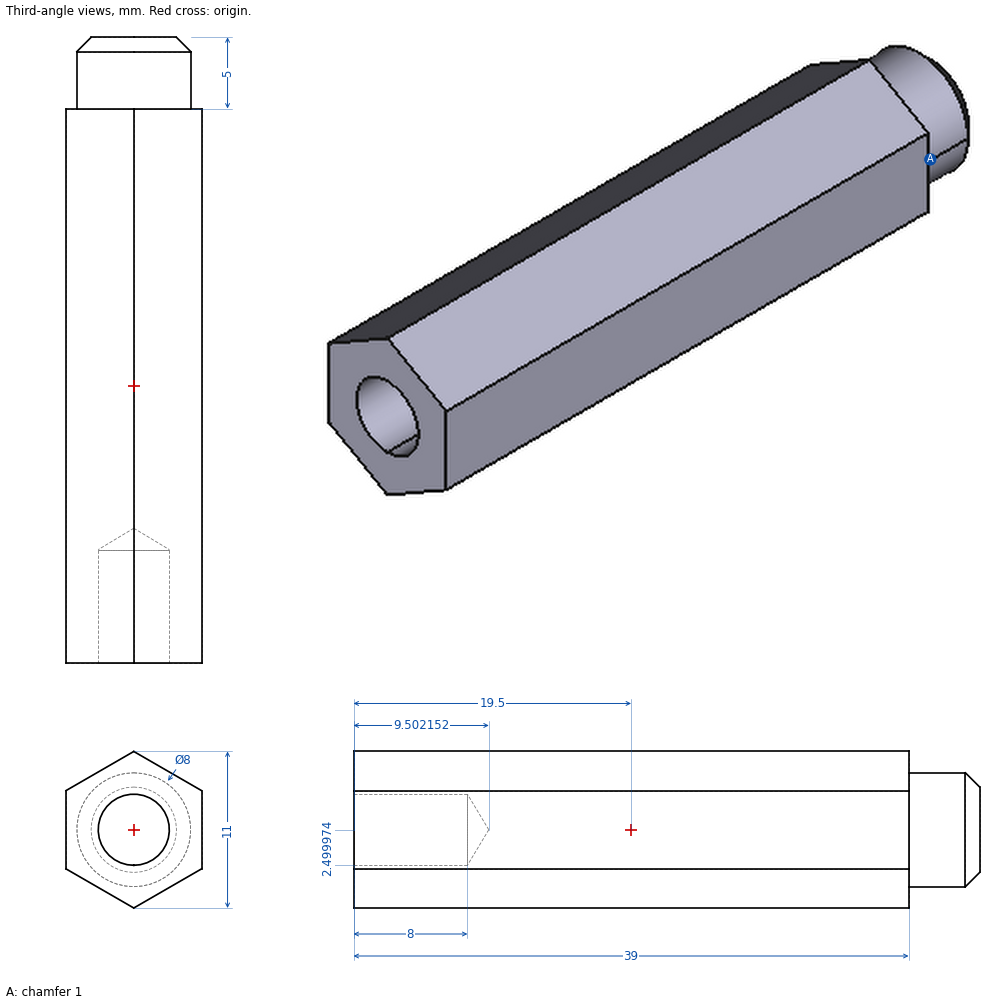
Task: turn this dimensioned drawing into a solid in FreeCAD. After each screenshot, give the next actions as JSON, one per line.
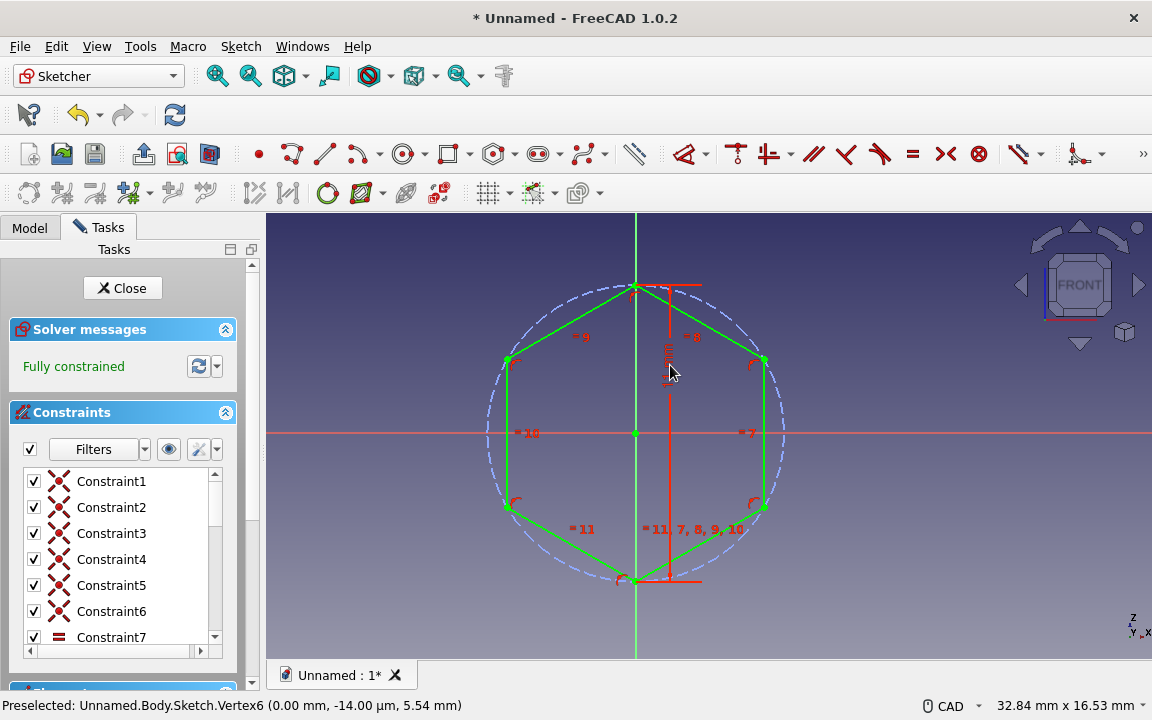
{"action": "left_click", "coordinate": [123, 288]}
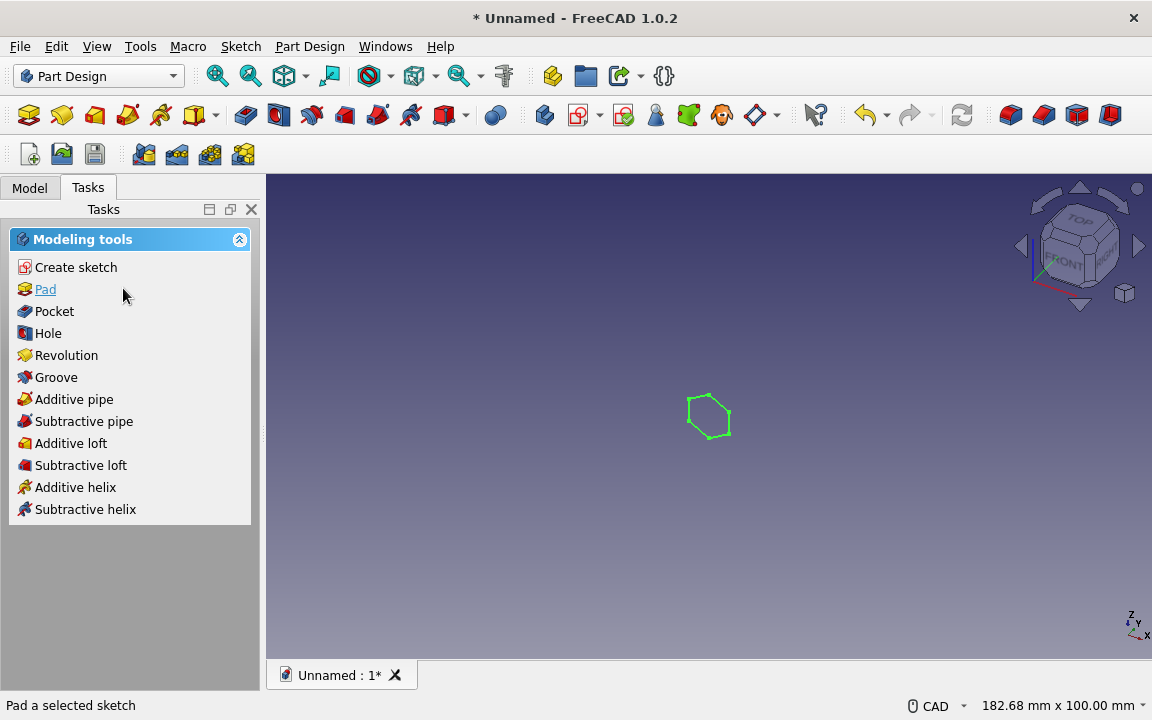
{"action": "left_click", "coordinate": [29, 116]}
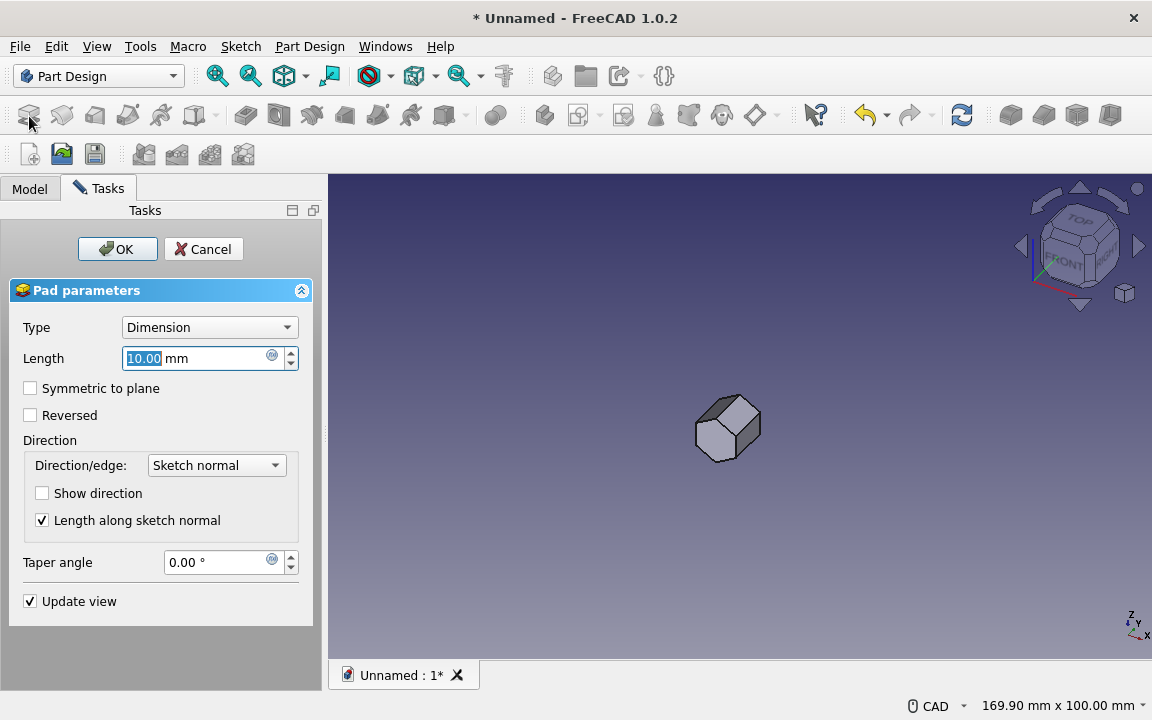
{"action": "type", "text": "39"}
{"action": "key", "text": "Tab"}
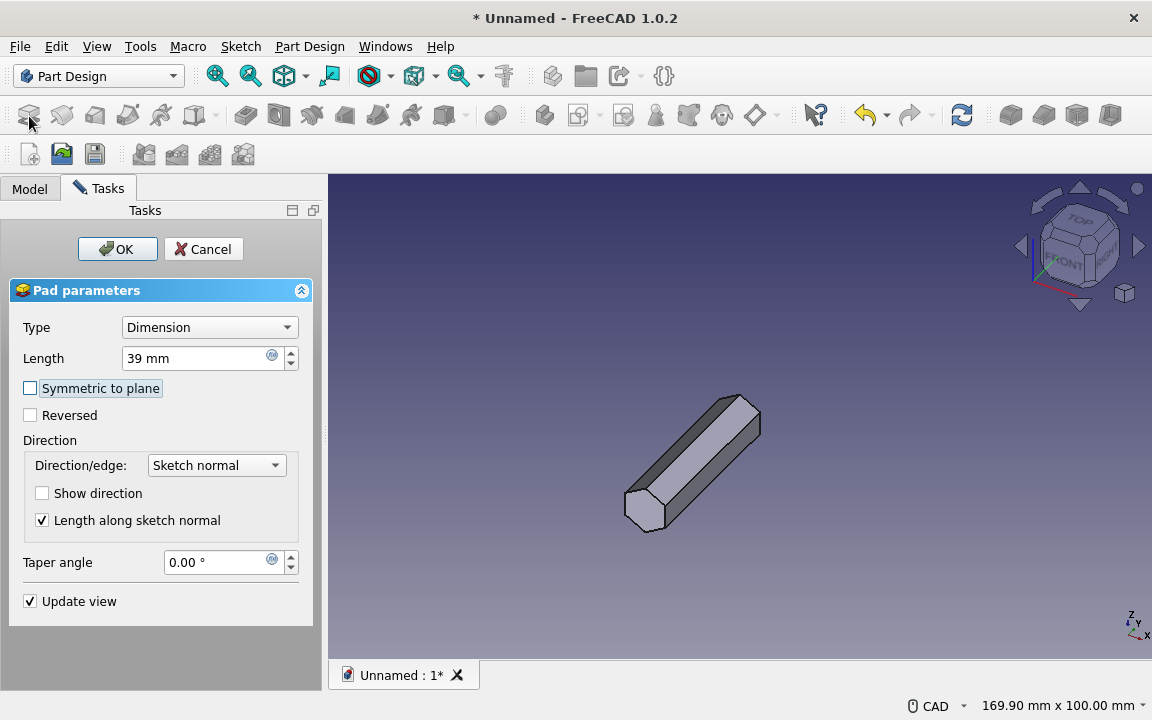
{"action": "left_click", "coordinate": [31, 388]}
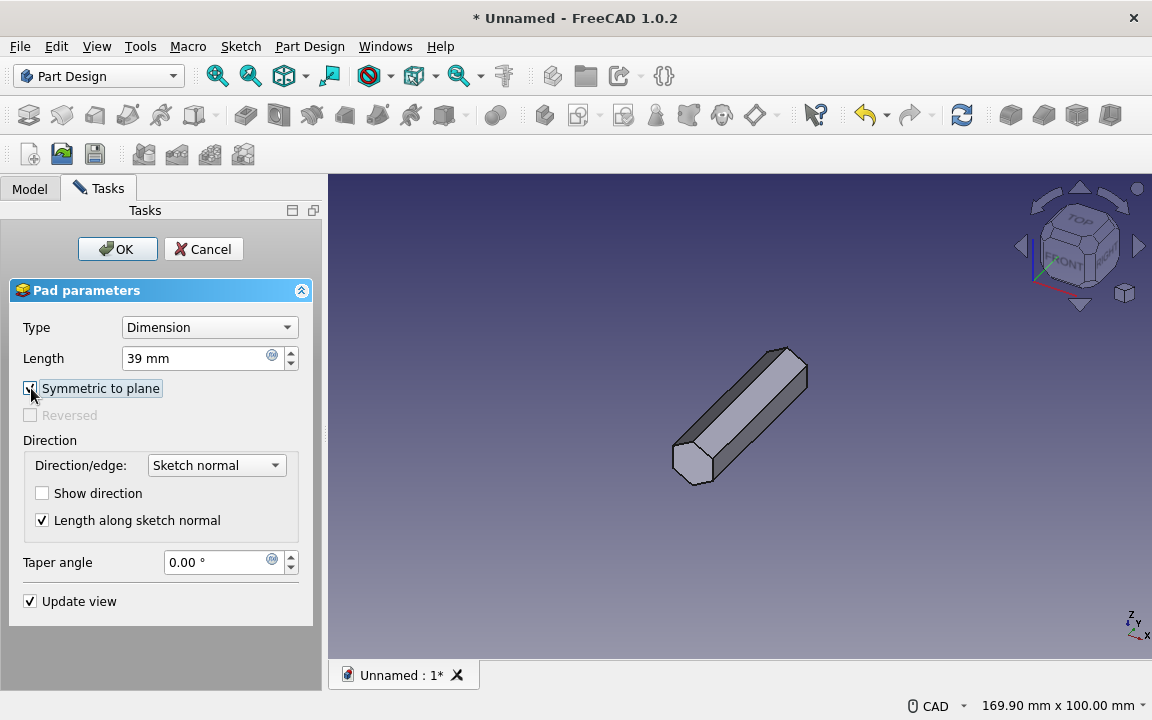
{"action": "left_click", "coordinate": [118, 249]}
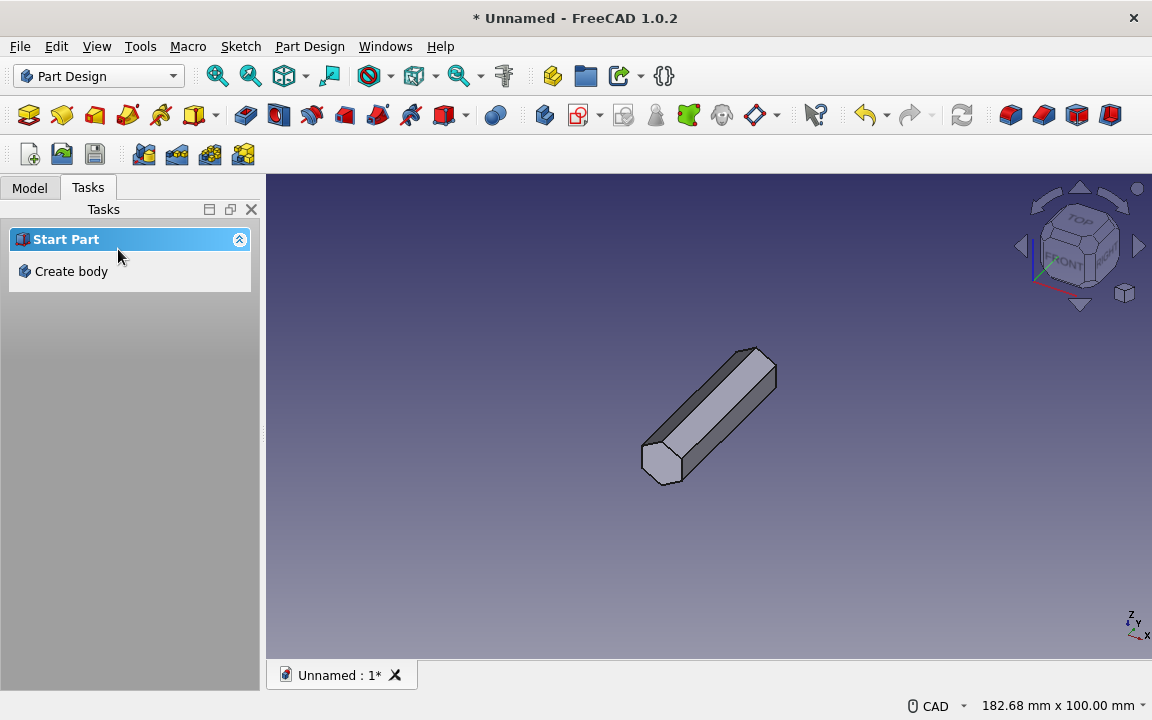
{"action": "left_click", "coordinate": [218, 76]}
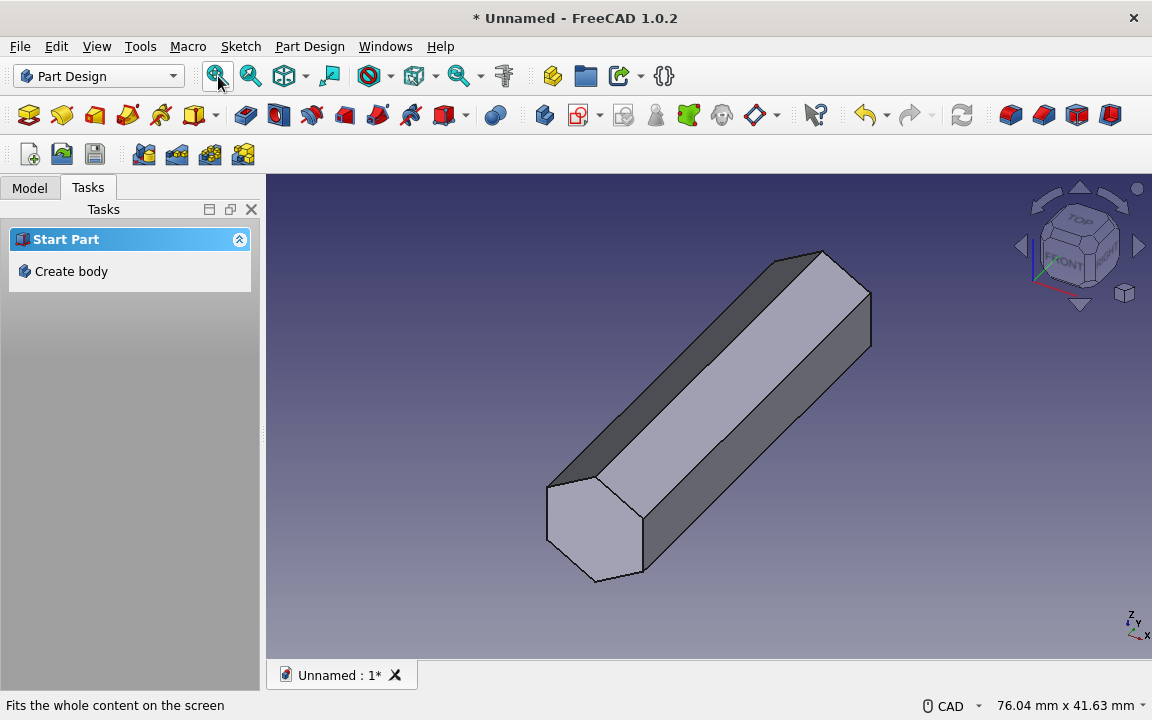
{"action": "key", "text": "4"}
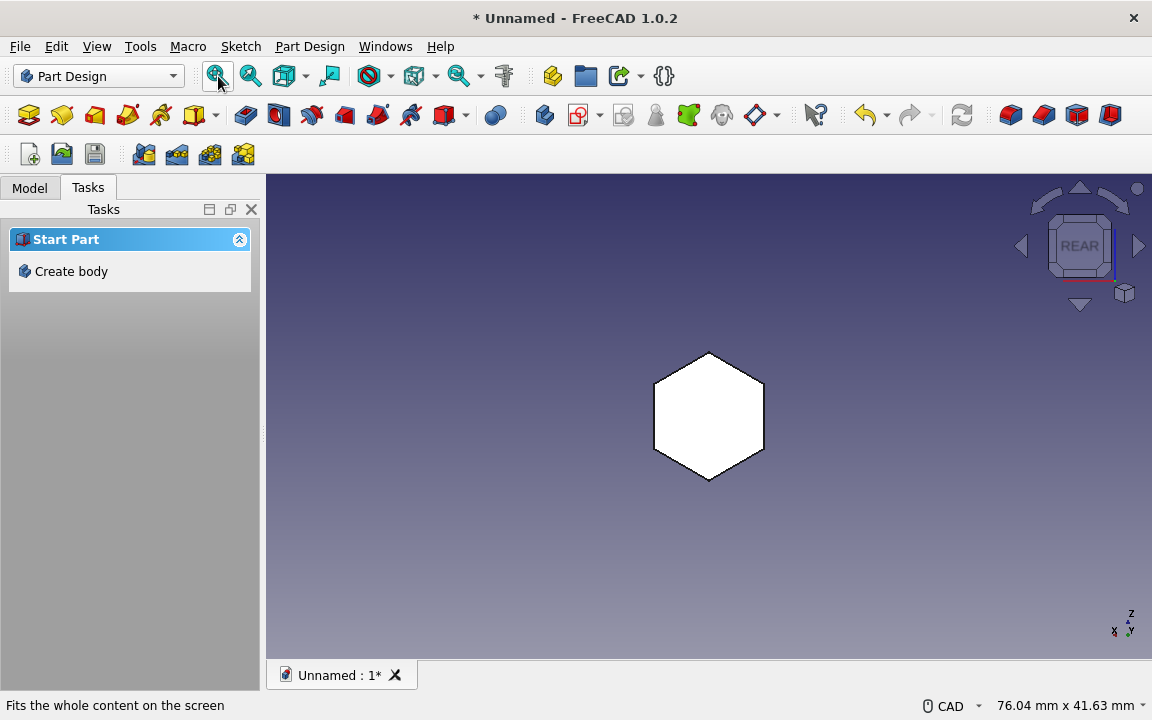
{"action": "left_click", "coordinate": [218, 76]}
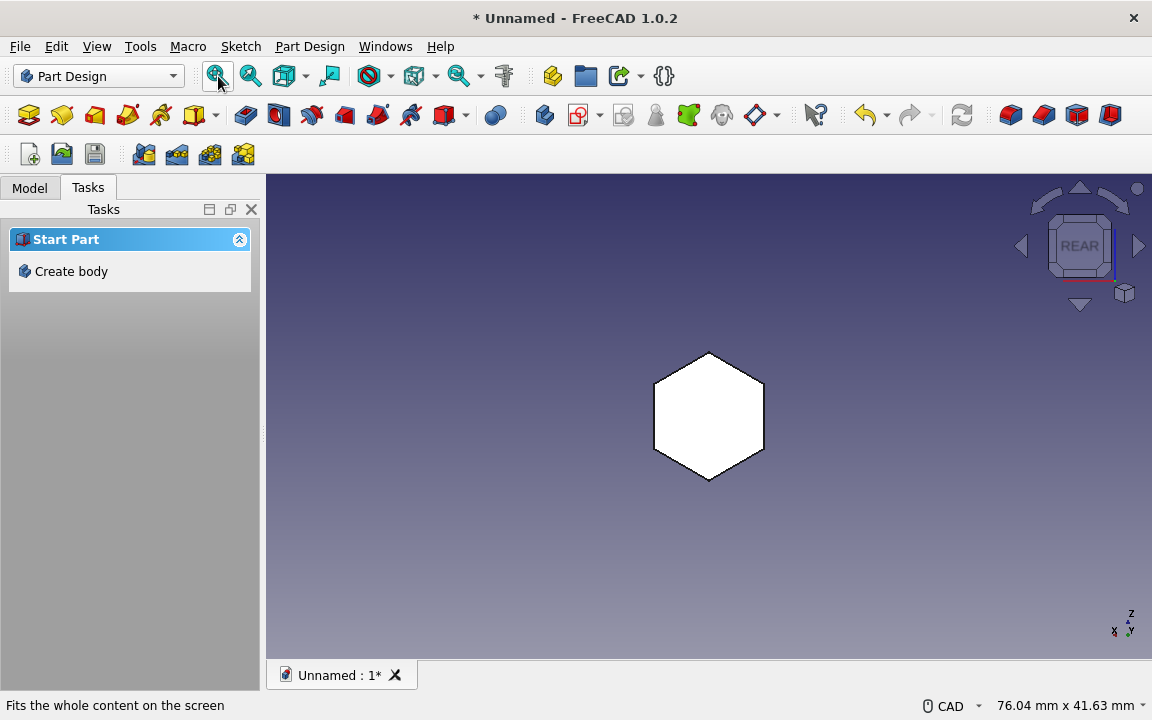
{"action": "left_click", "coordinate": [709, 416]}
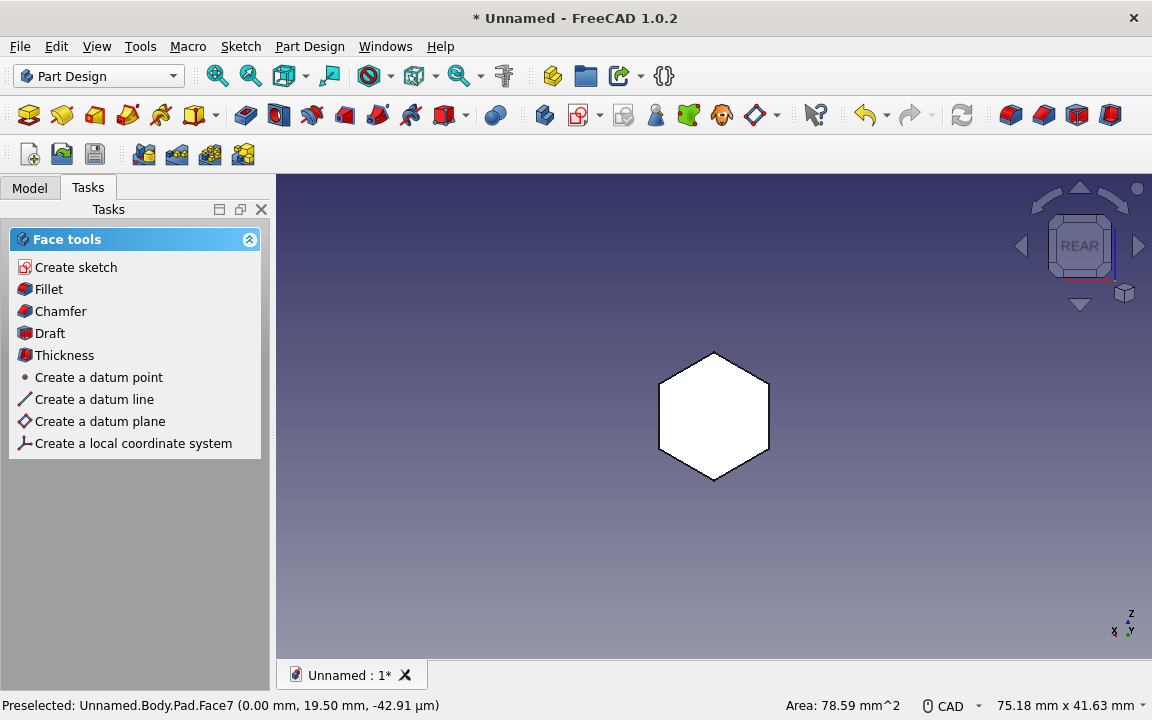
{"action": "left_click", "coordinate": [578, 116]}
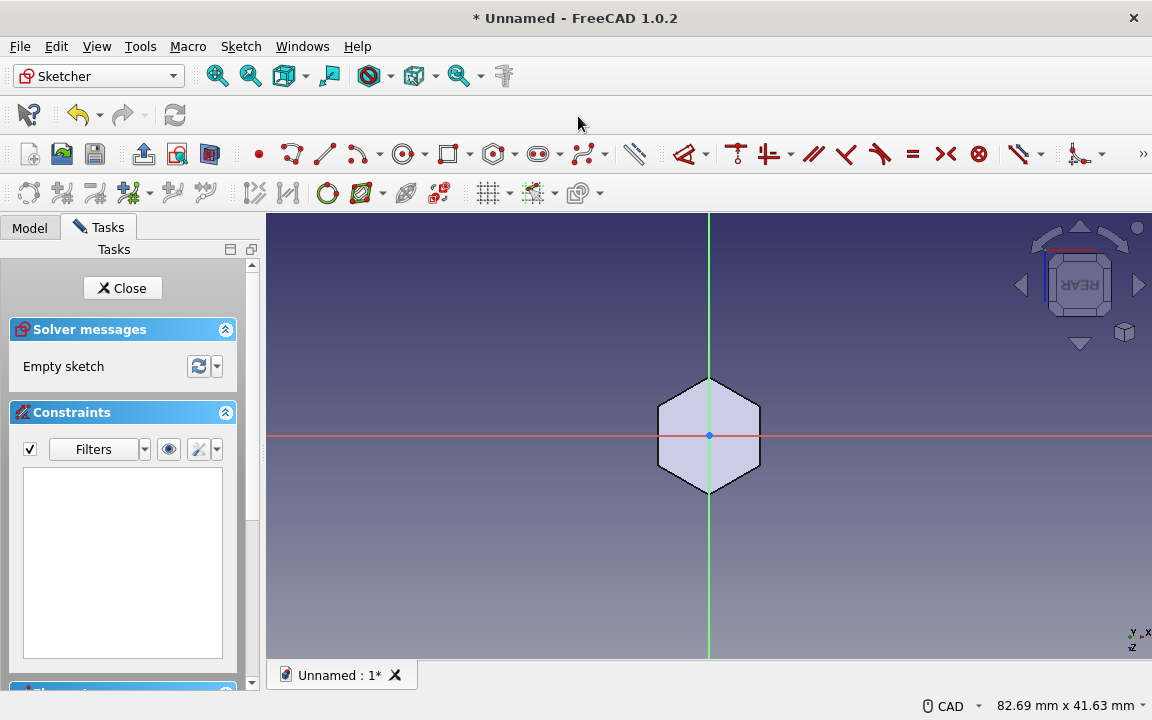
{"action": "scroll", "coordinate": [739, 436], "scroll_direction": "up", "scroll_amount": 6}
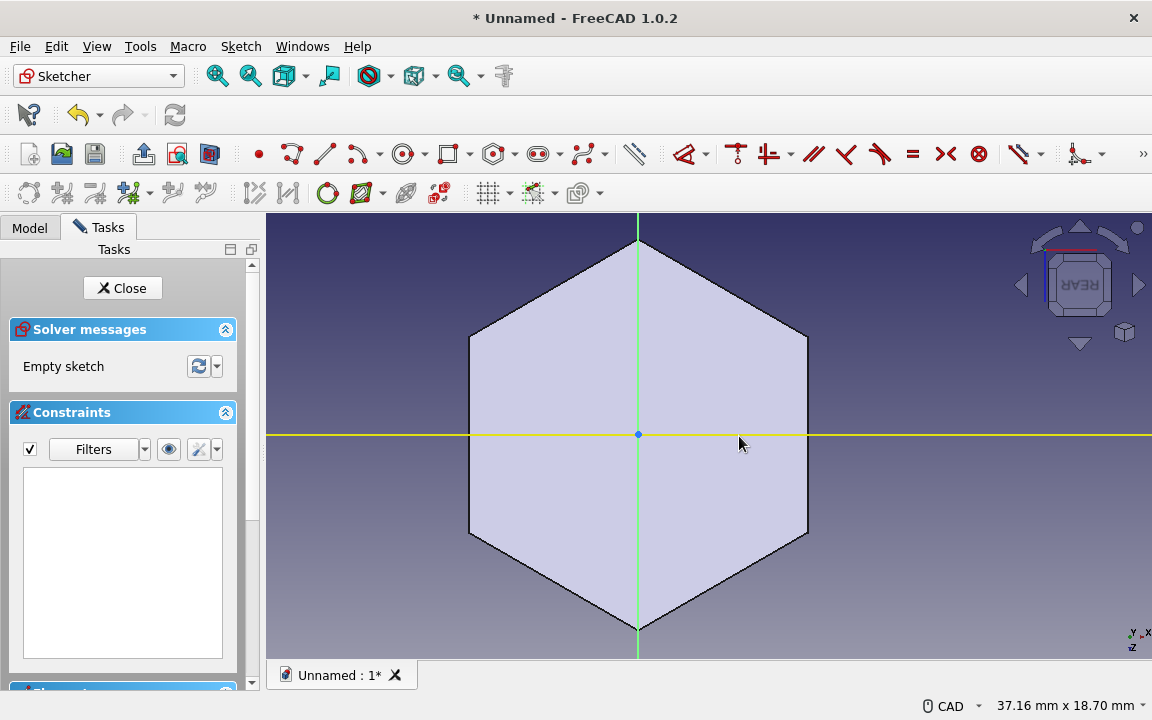
{"action": "left_click", "coordinate": [402, 154]}